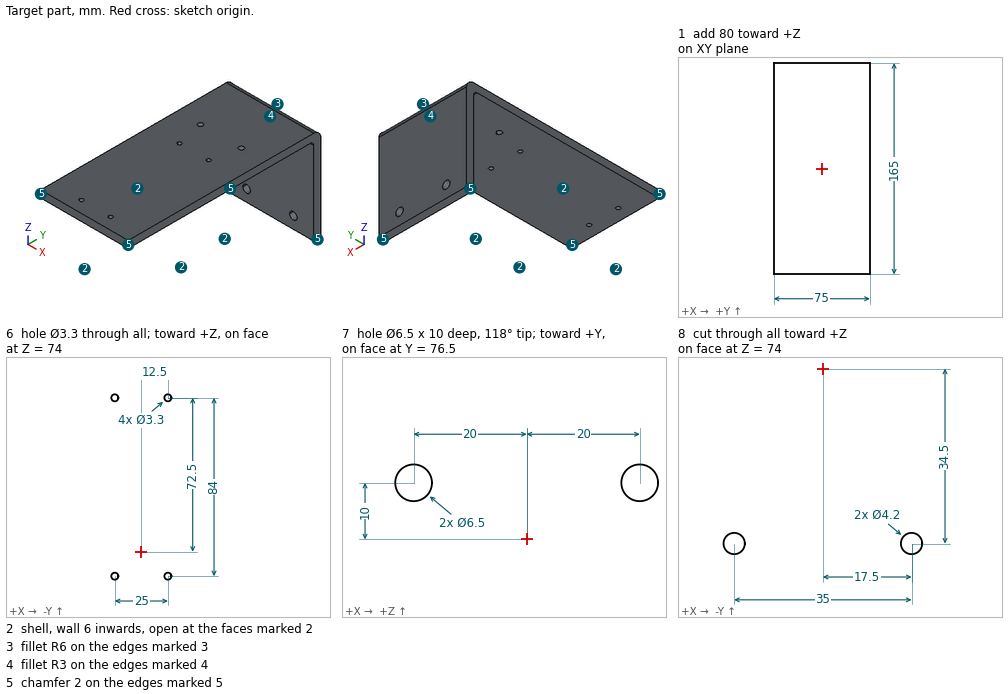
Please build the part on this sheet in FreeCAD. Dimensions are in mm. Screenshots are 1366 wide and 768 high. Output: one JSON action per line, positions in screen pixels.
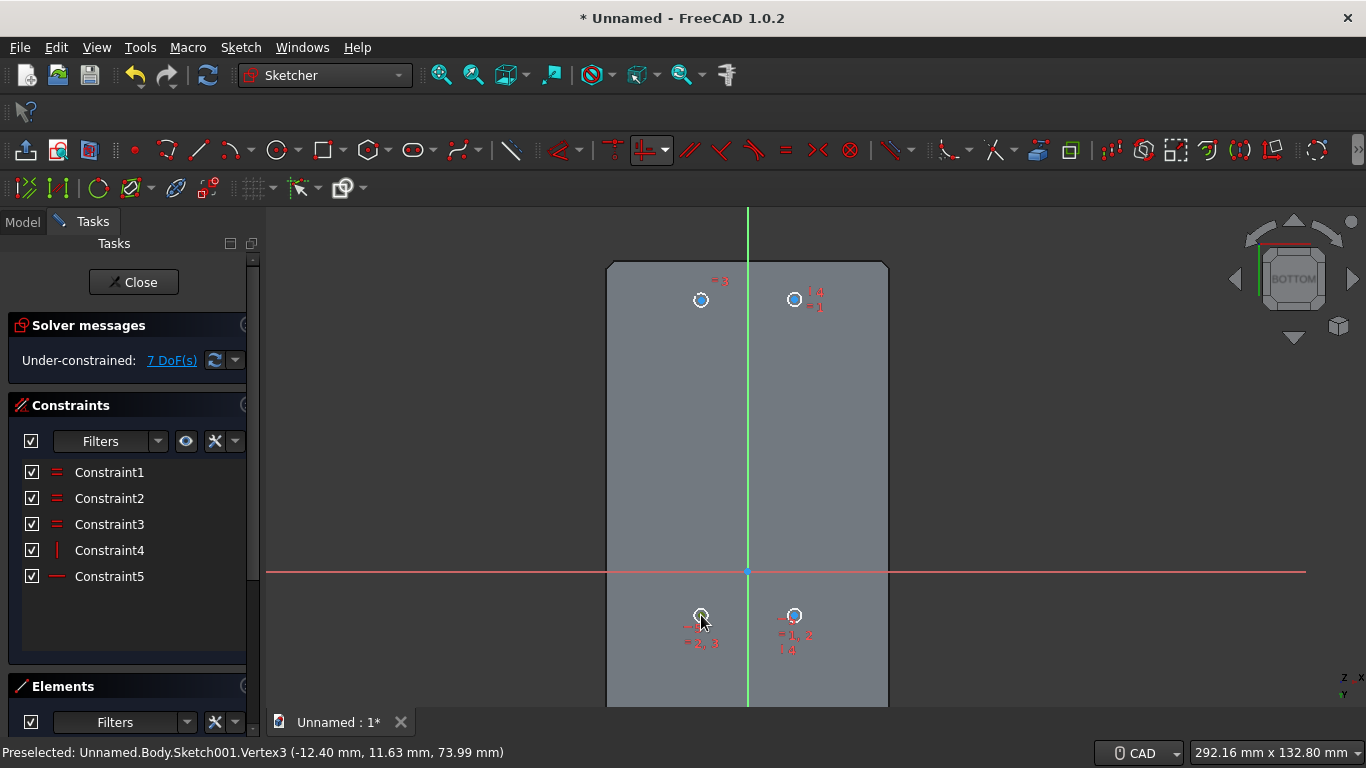
{"action": "left_click", "coordinate": [701, 300]}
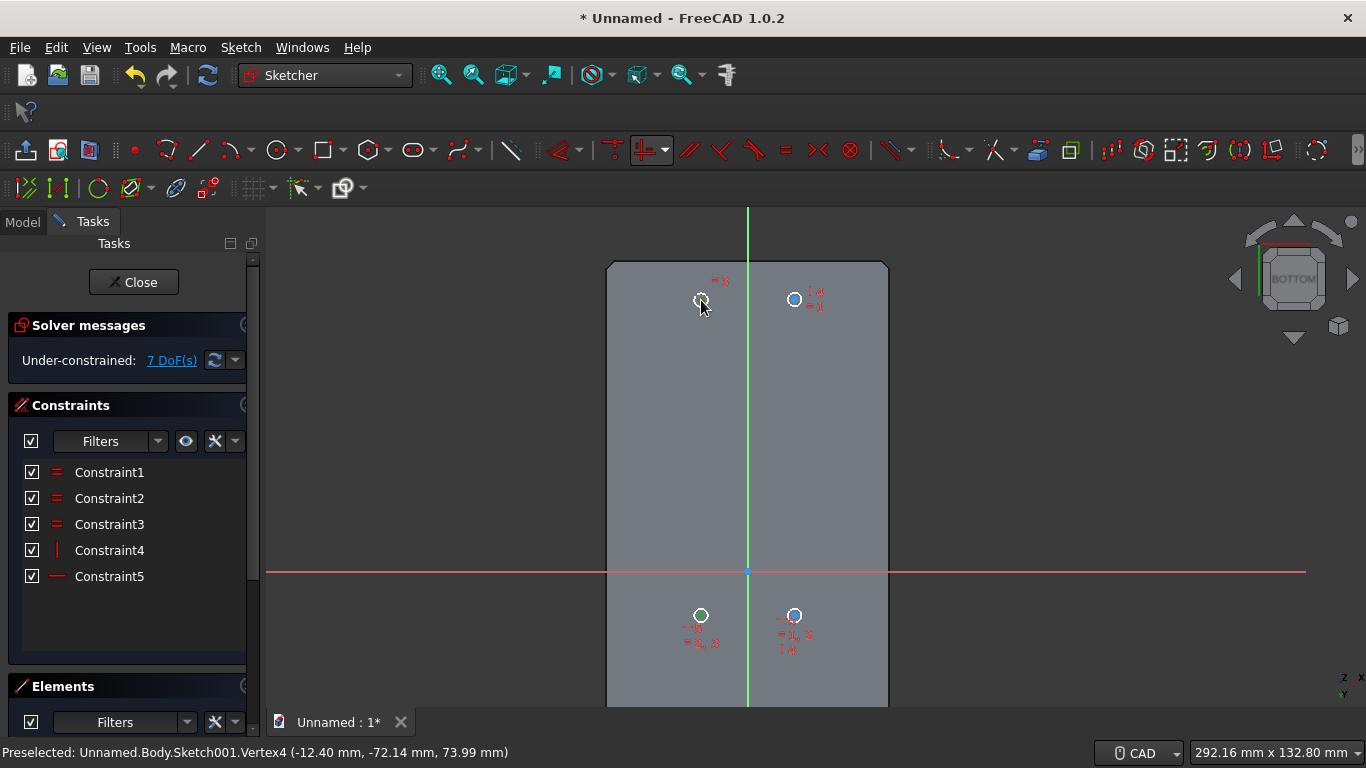
{"action": "left_click", "coordinate": [668, 150]}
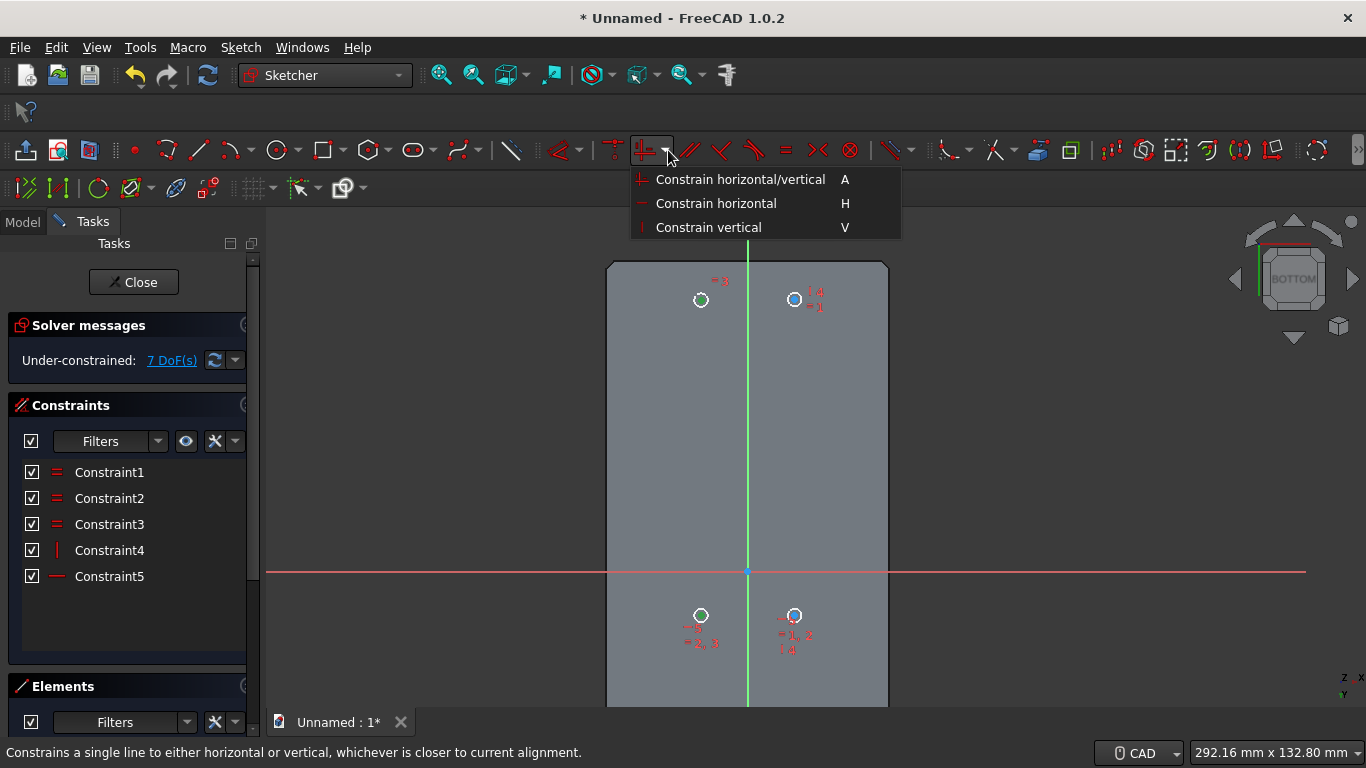
{"action": "left_click", "coordinate": [766, 227]}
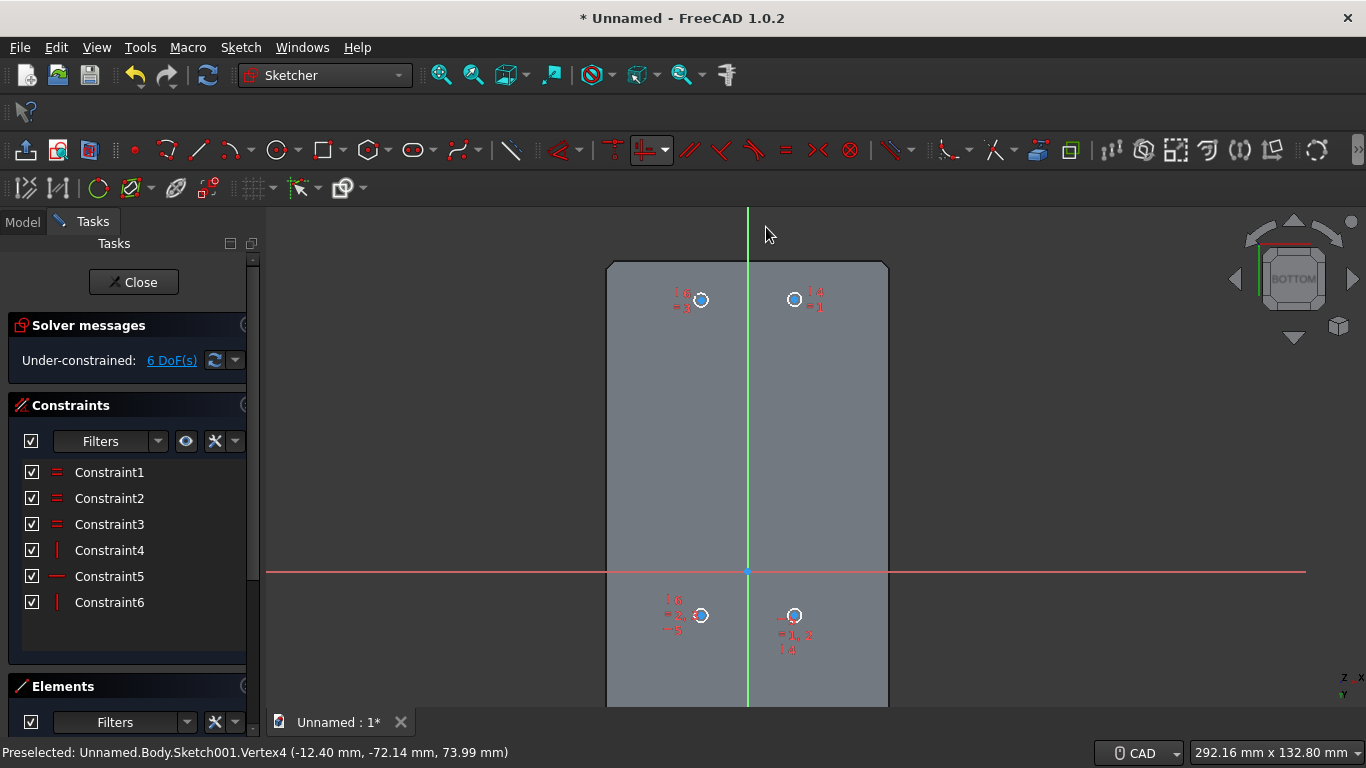
{"action": "left_click", "coordinate": [795, 299]}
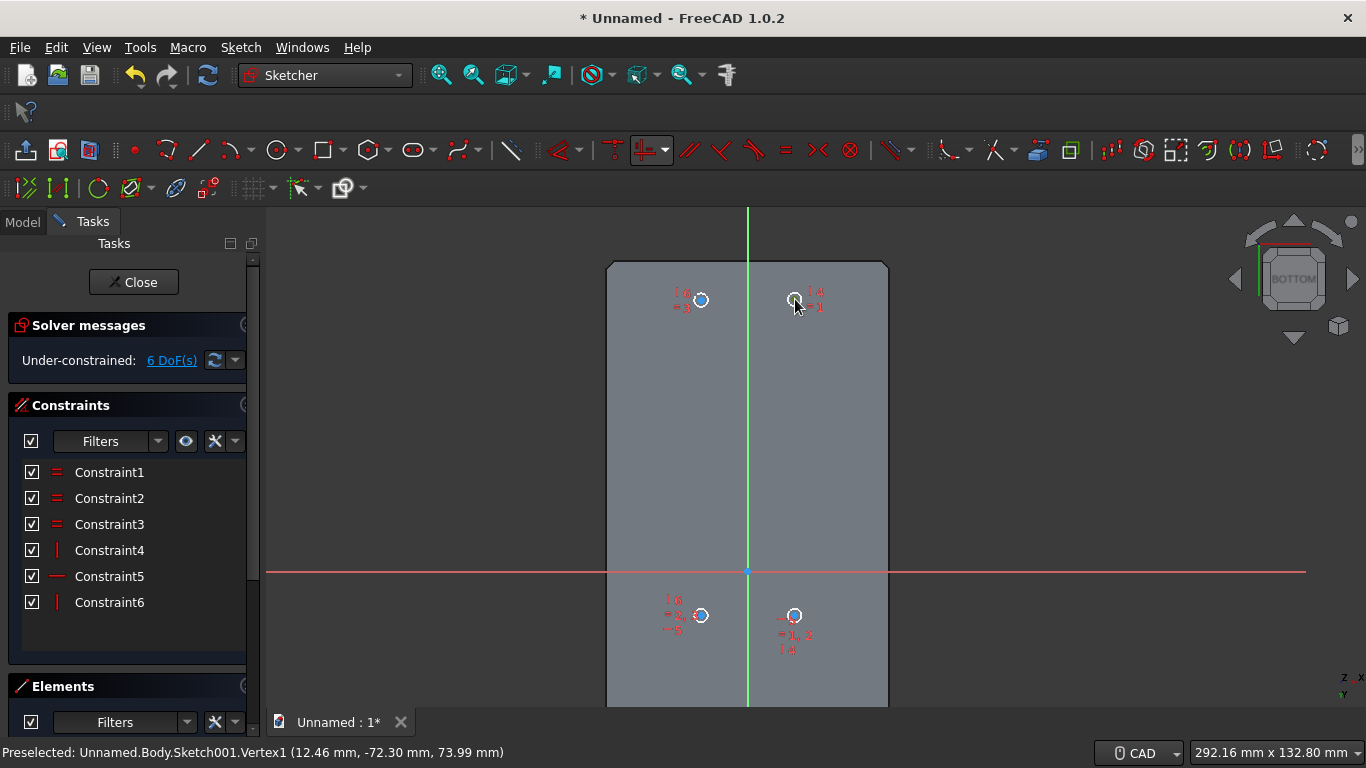
{"action": "left_click", "coordinate": [701, 300]}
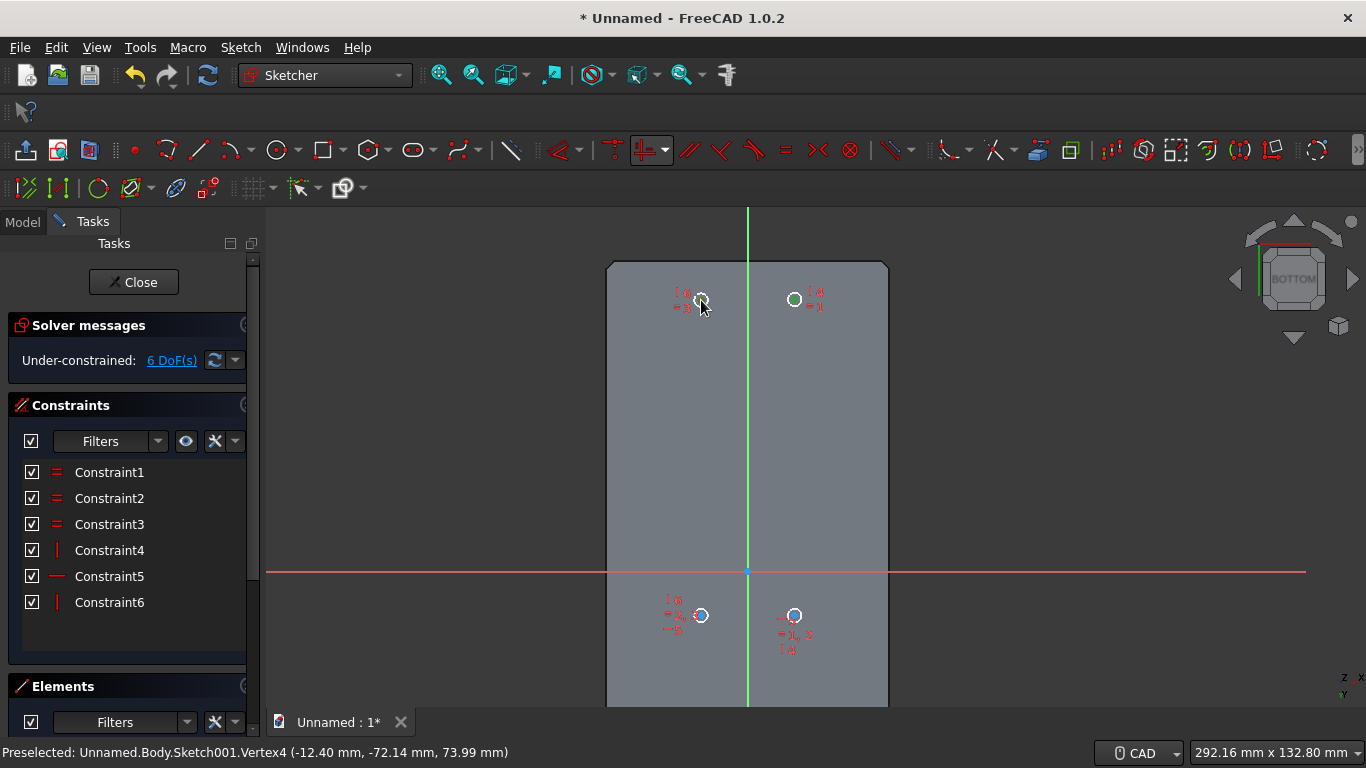
{"action": "left_click", "coordinate": [668, 150]}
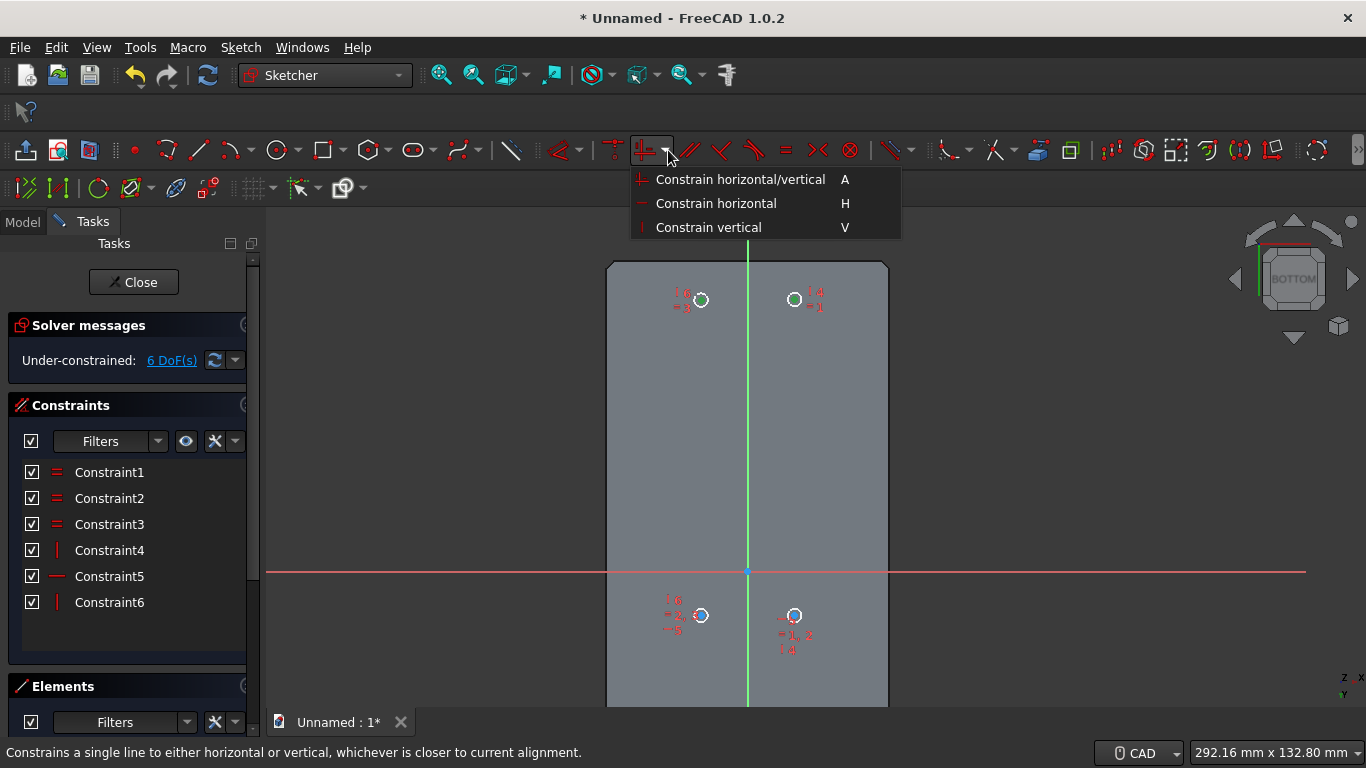
{"action": "left_click", "coordinate": [766, 203]}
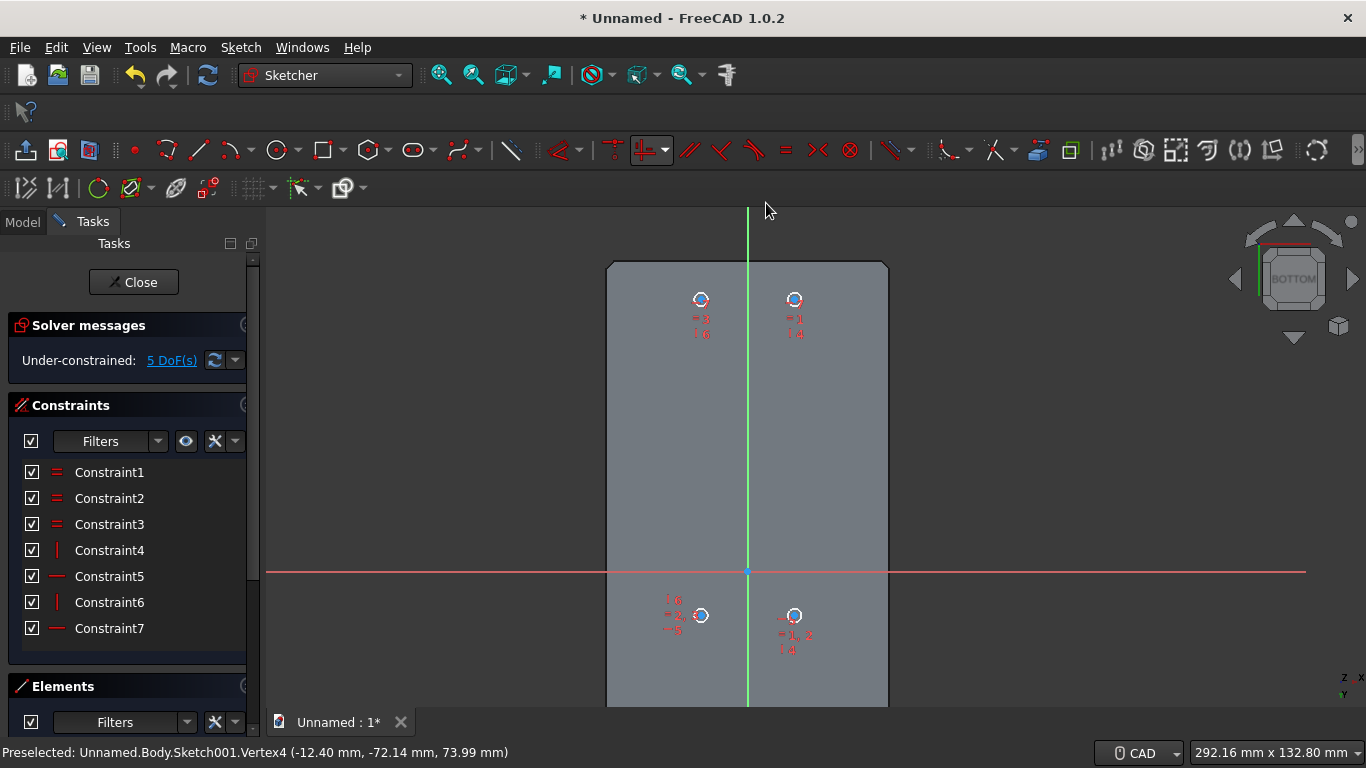
{"action": "left_click", "coordinate": [558, 150]}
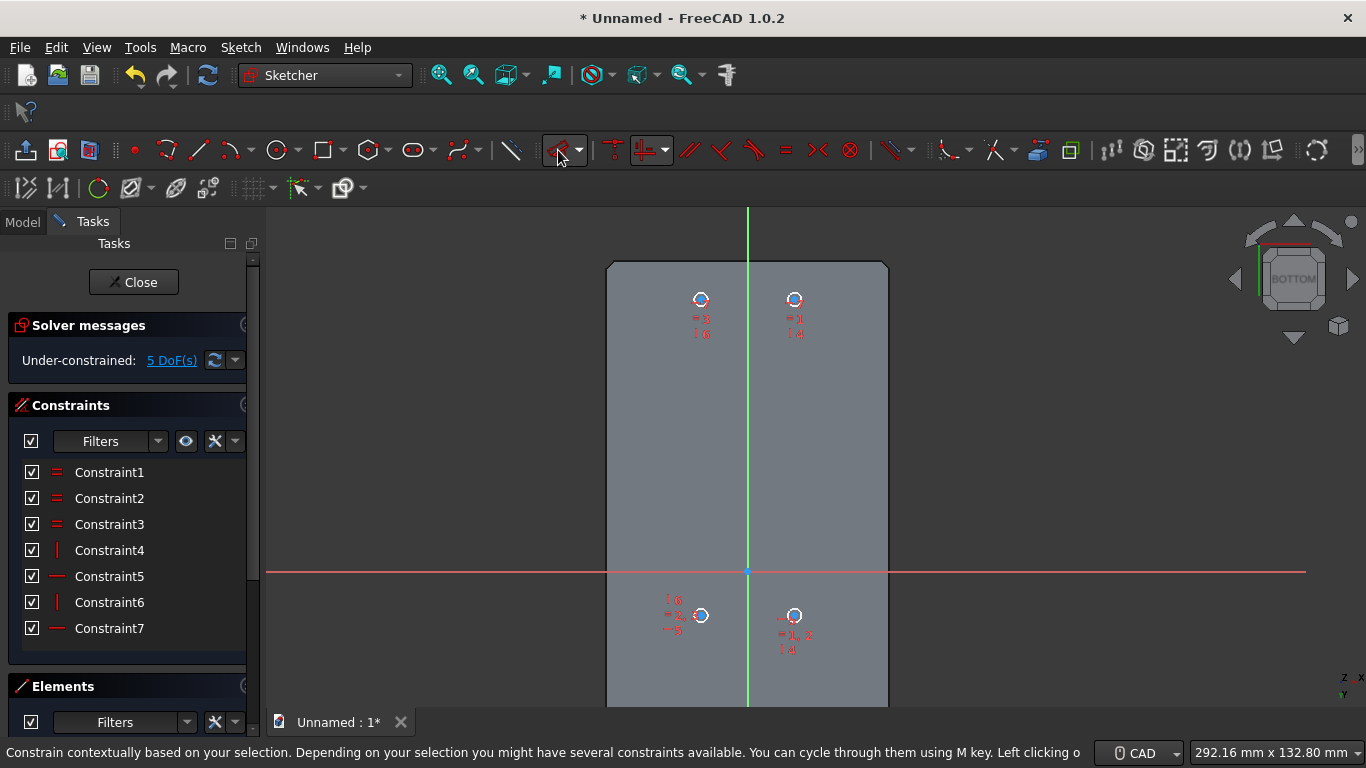
{"action": "scroll", "coordinate": [795, 293], "scroll_direction": "up", "scroll_amount": 6}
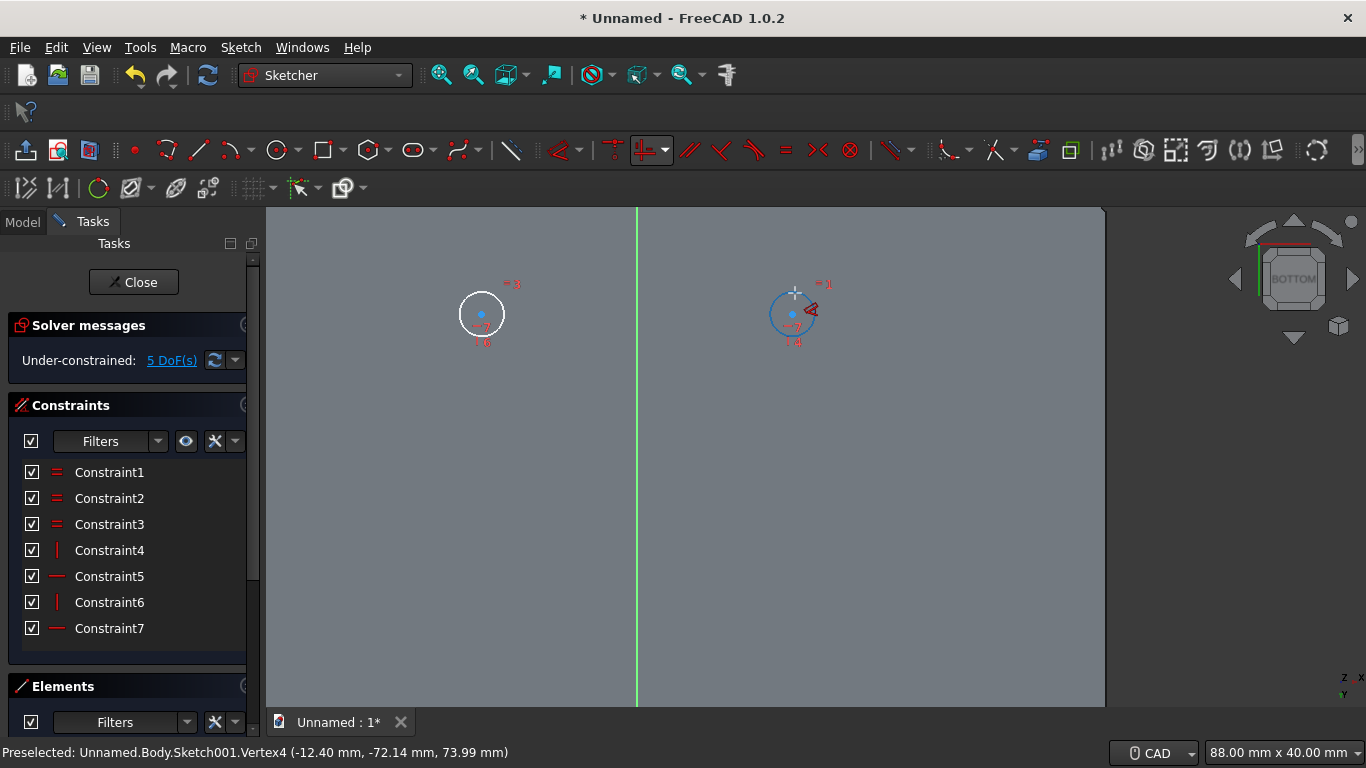
{"action": "left_click", "coordinate": [793, 292]}
{"action": "left_click", "coordinate": [794, 260]}